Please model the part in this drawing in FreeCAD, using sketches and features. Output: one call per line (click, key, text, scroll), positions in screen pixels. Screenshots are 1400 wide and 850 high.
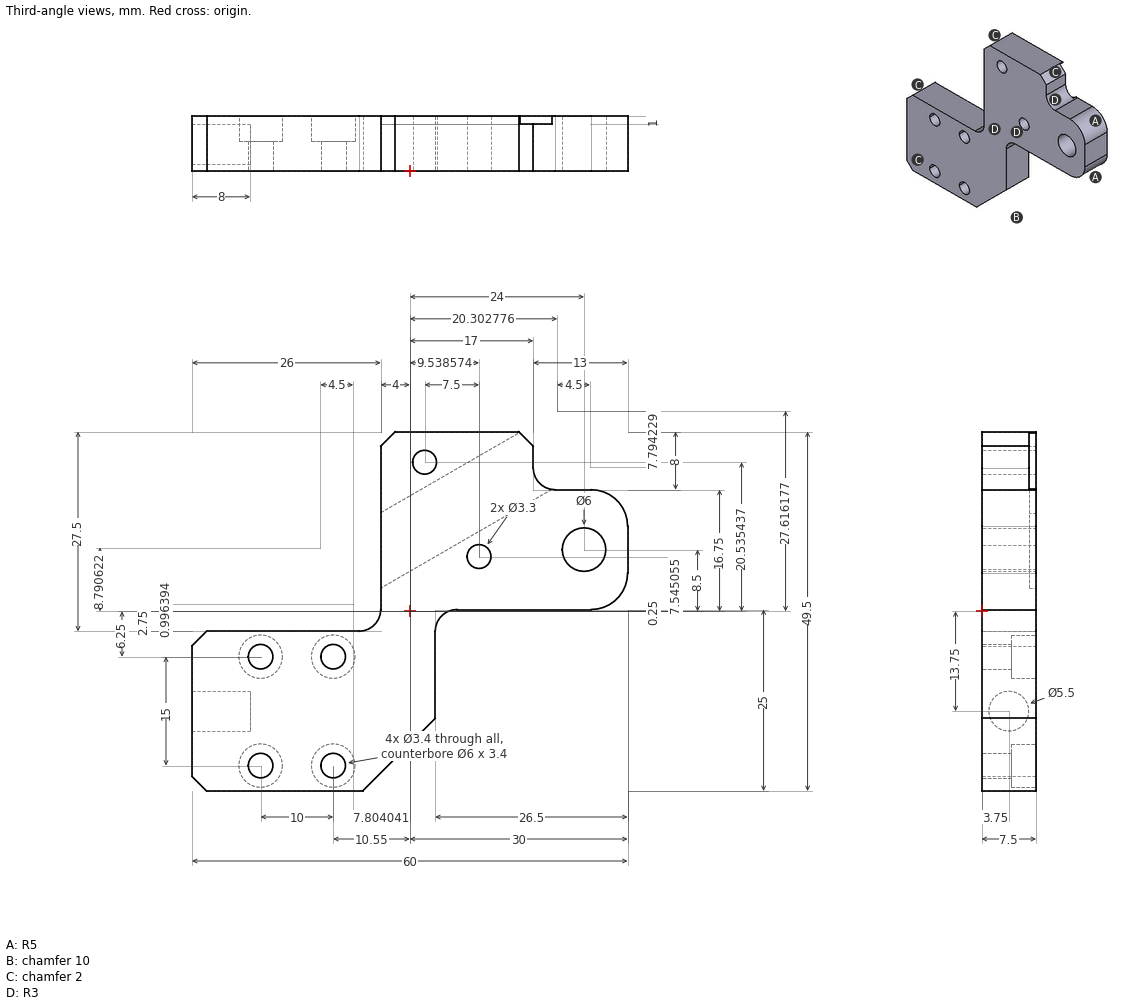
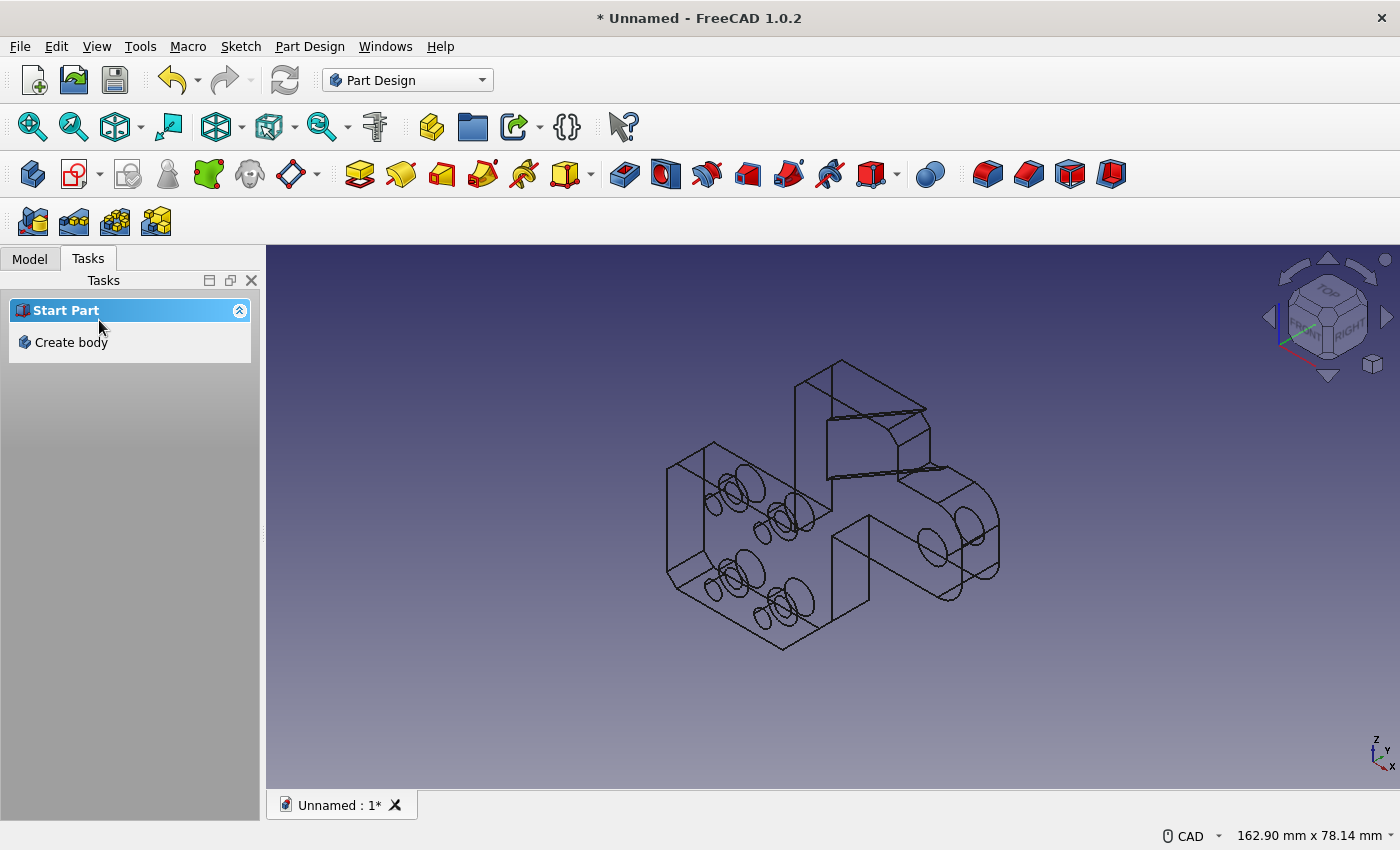
click(850, 525)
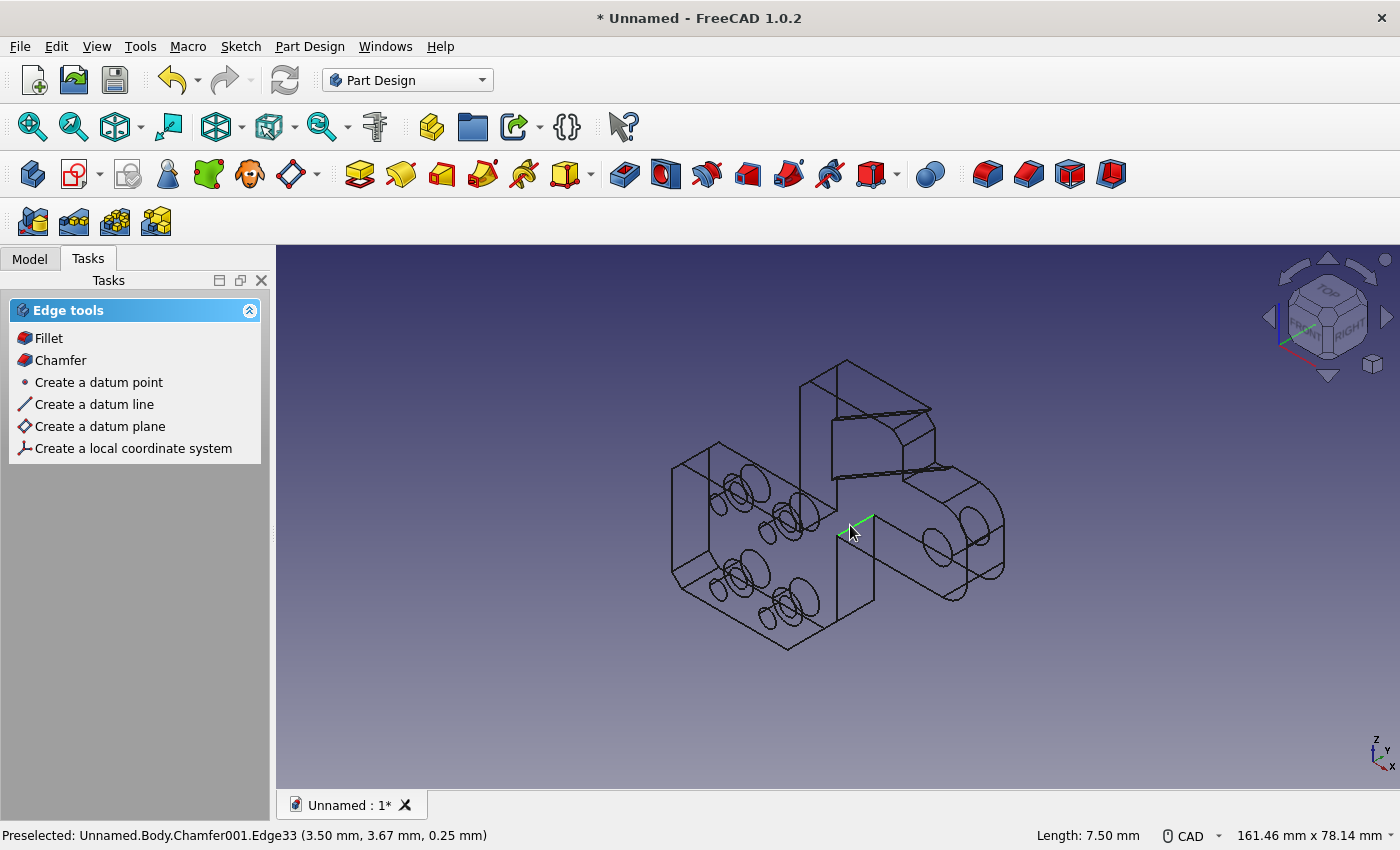
click(919, 471, ctrl)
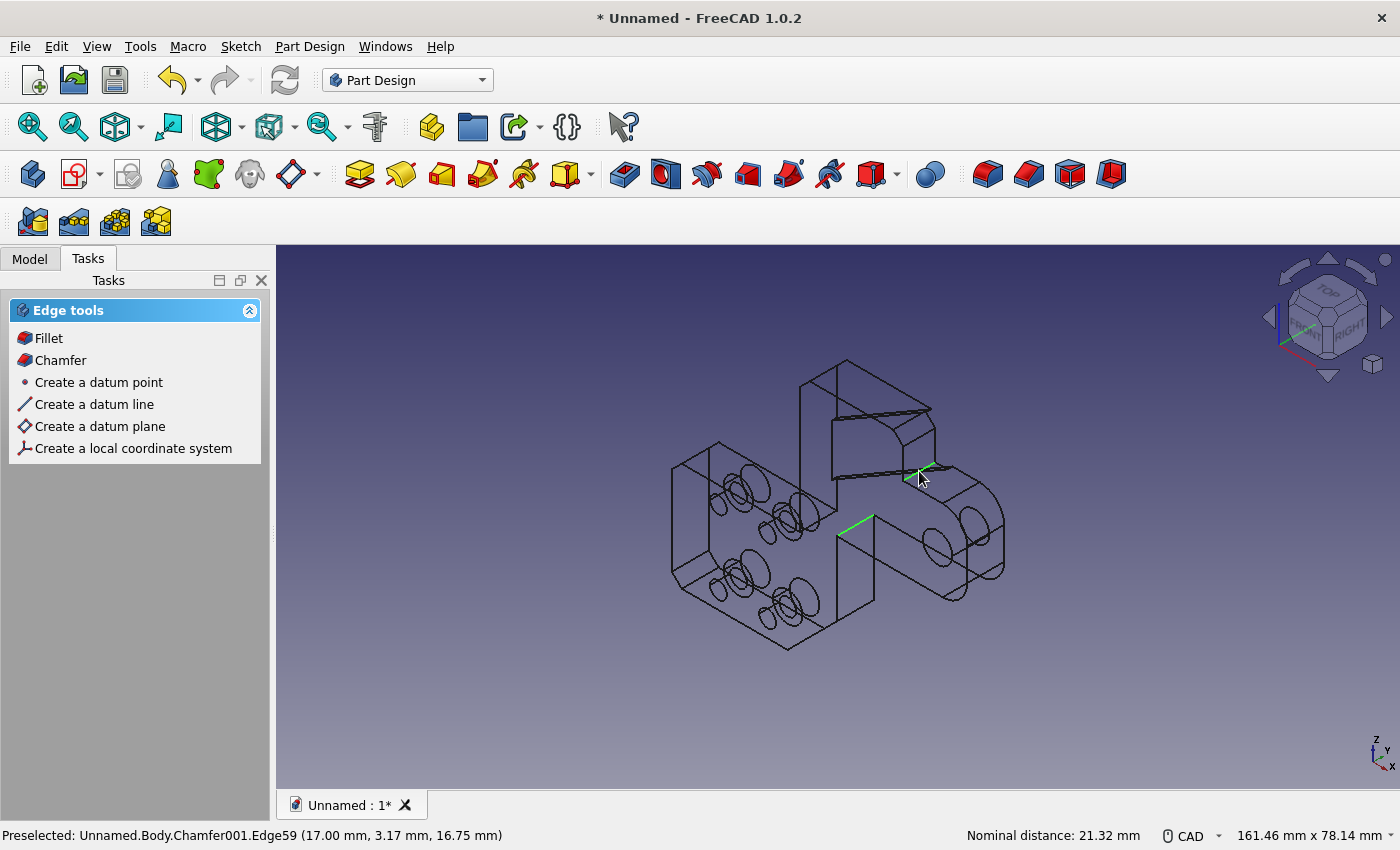
click(818, 520, ctrl)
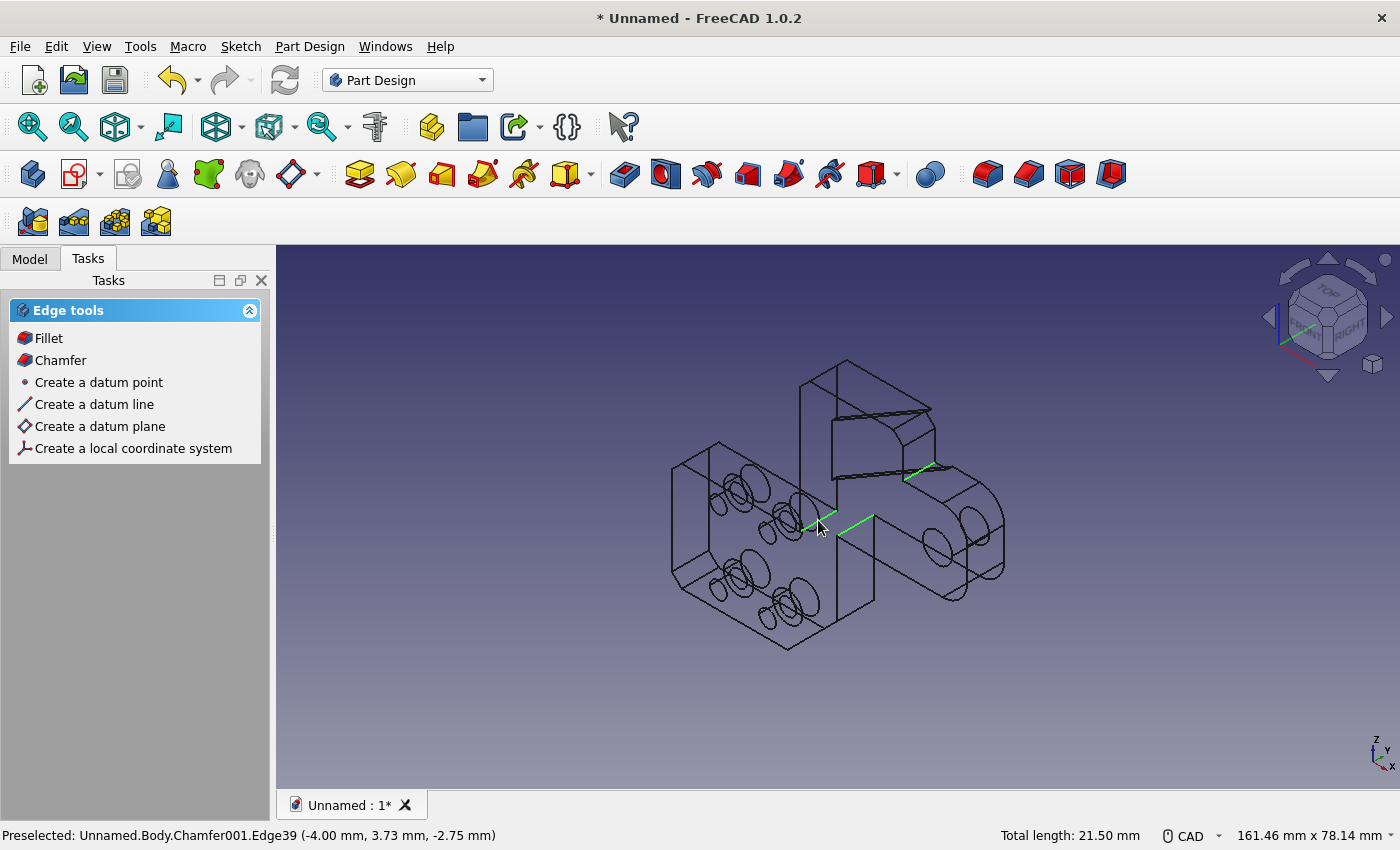
key(v)
key(1)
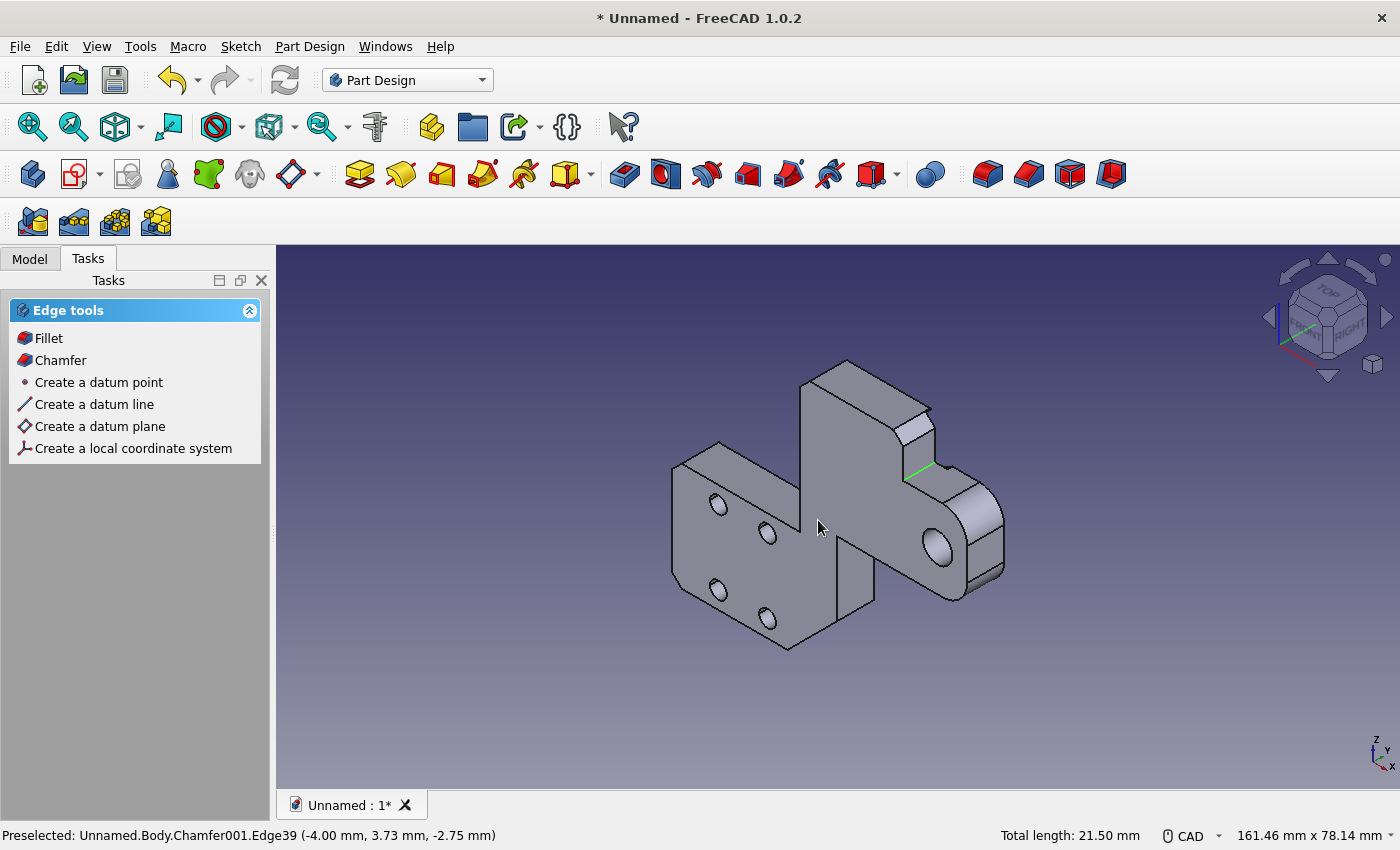
click(988, 174)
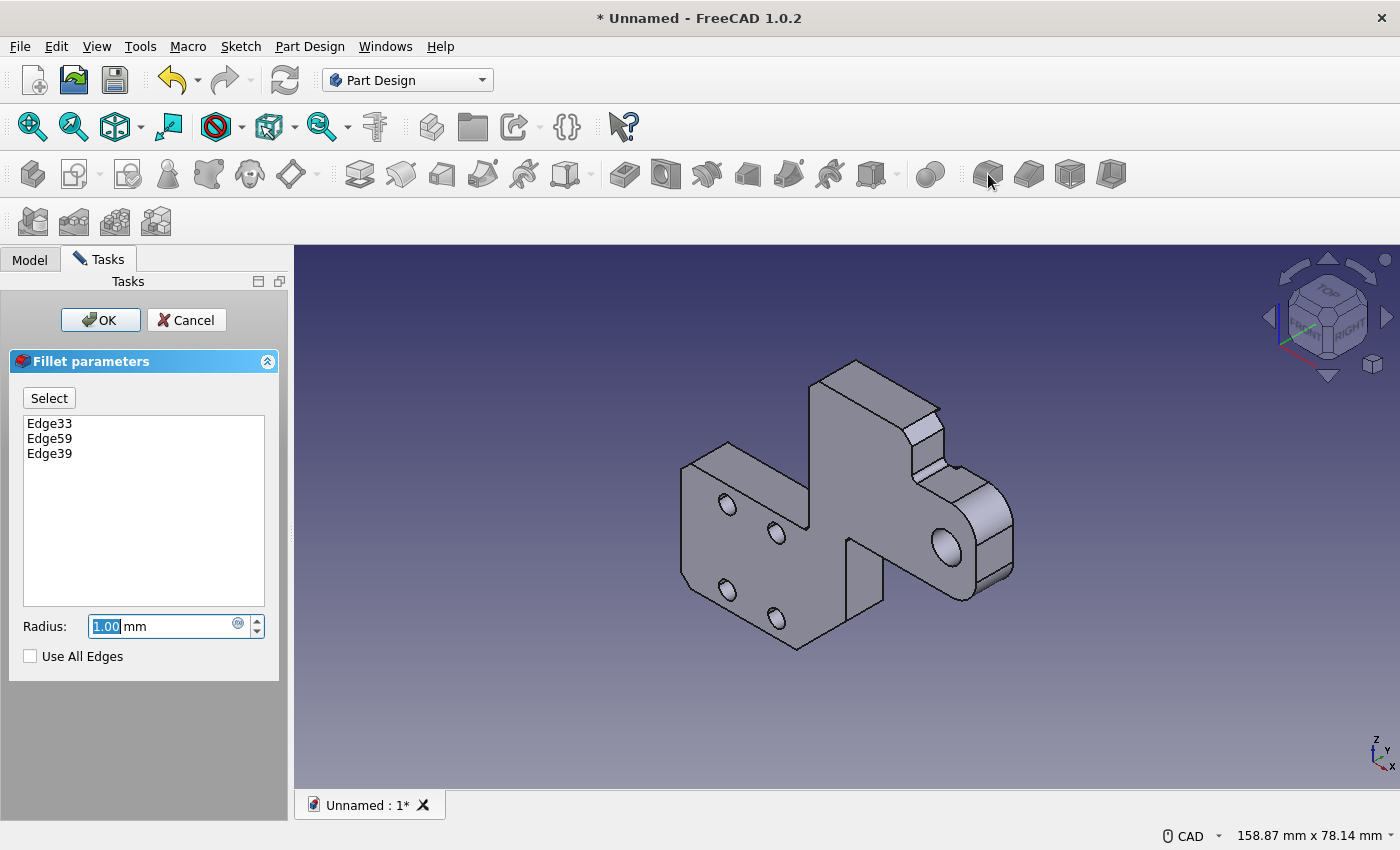
text(3)
key(Tab)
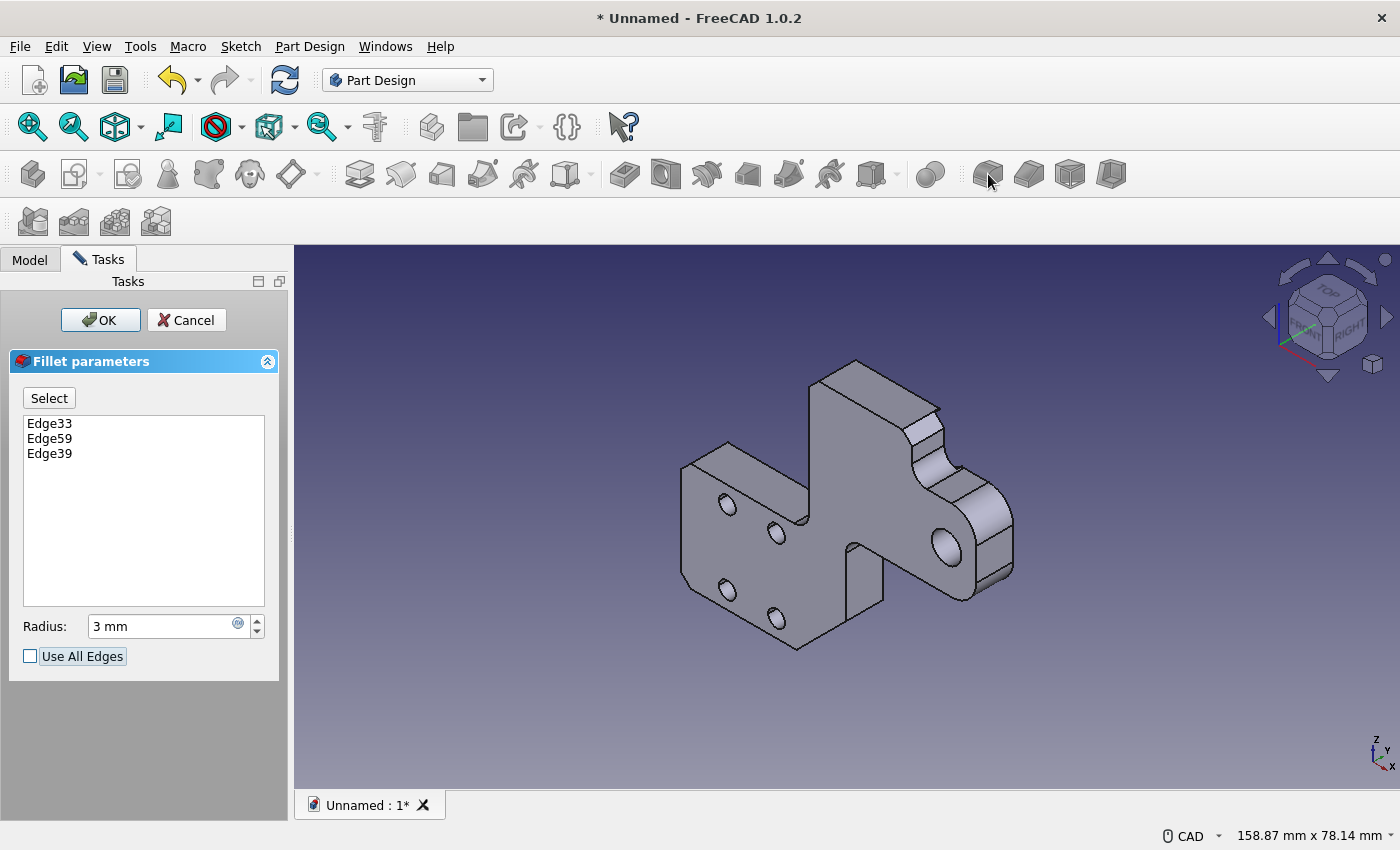
click(101, 320)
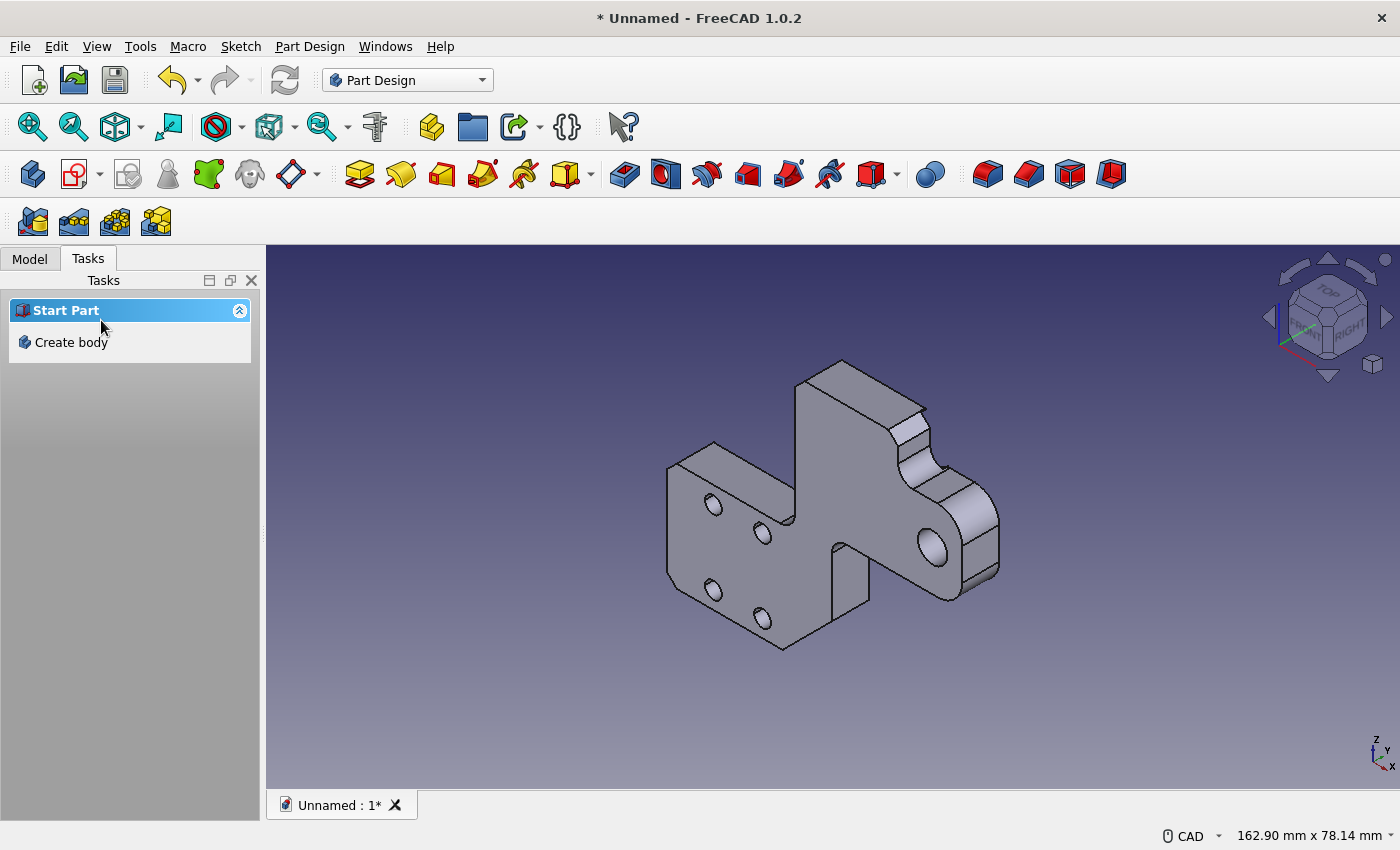
key(4)